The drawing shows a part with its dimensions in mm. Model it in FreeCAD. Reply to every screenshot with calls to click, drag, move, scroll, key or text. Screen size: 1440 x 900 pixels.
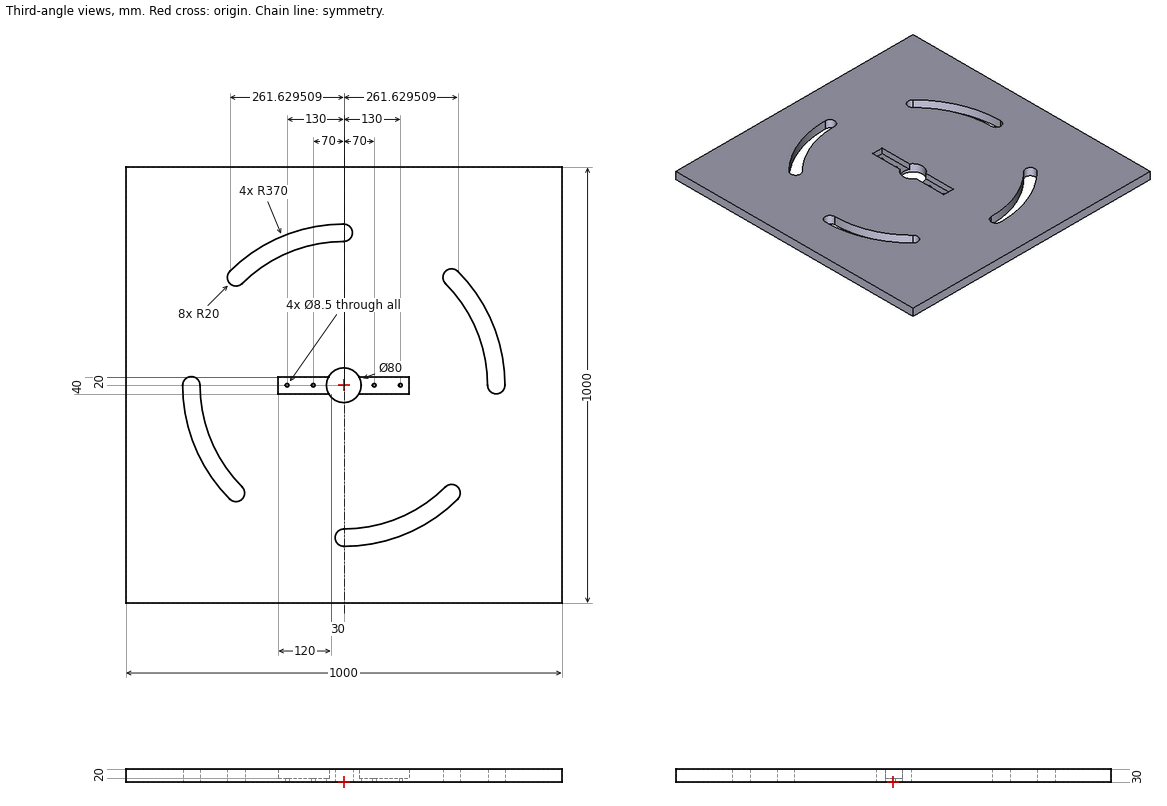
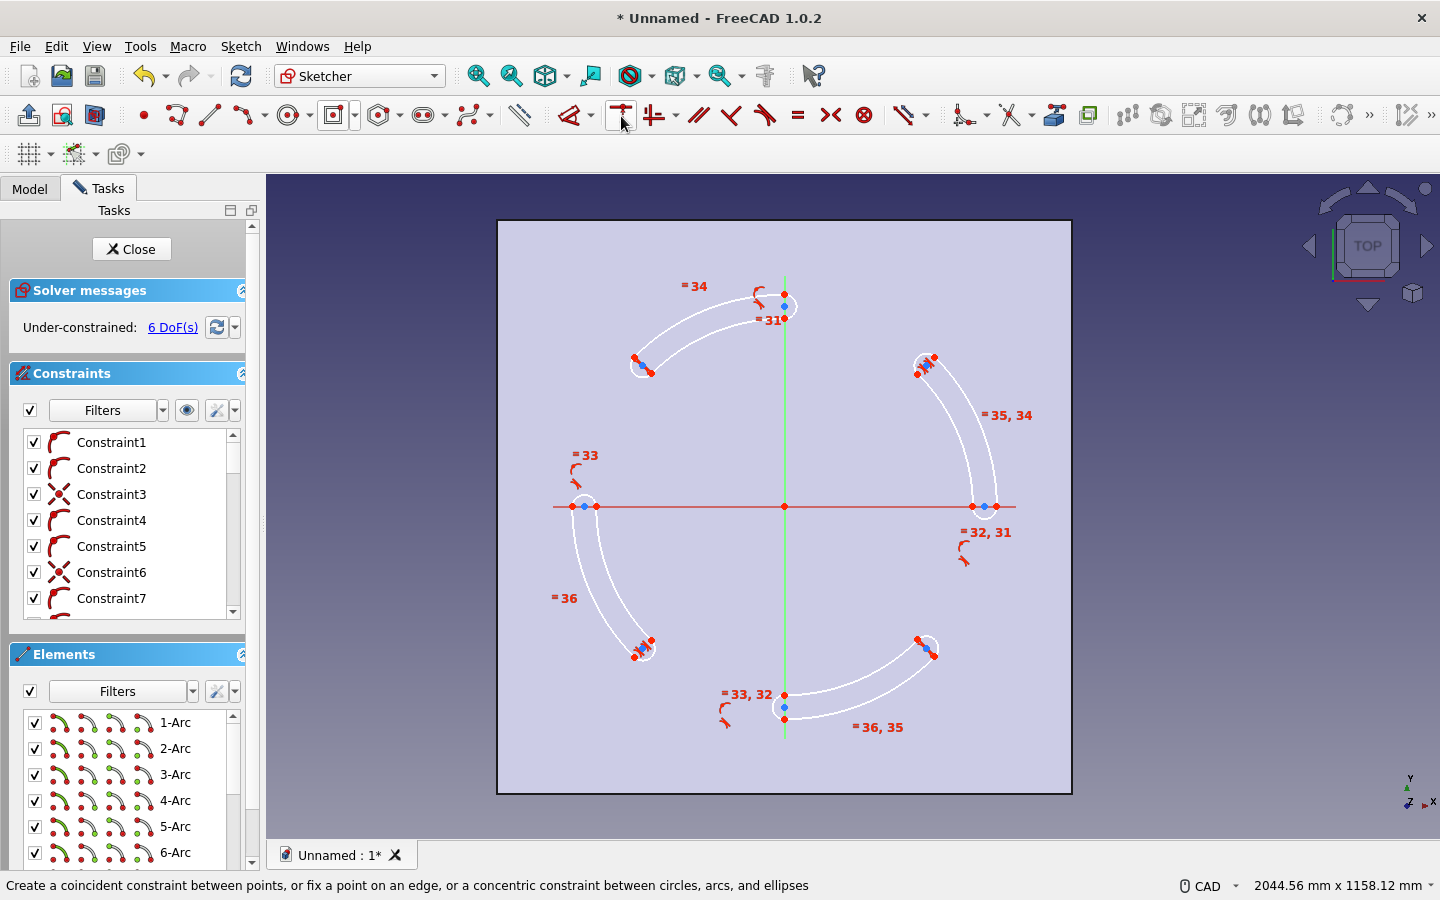
click(568, 116)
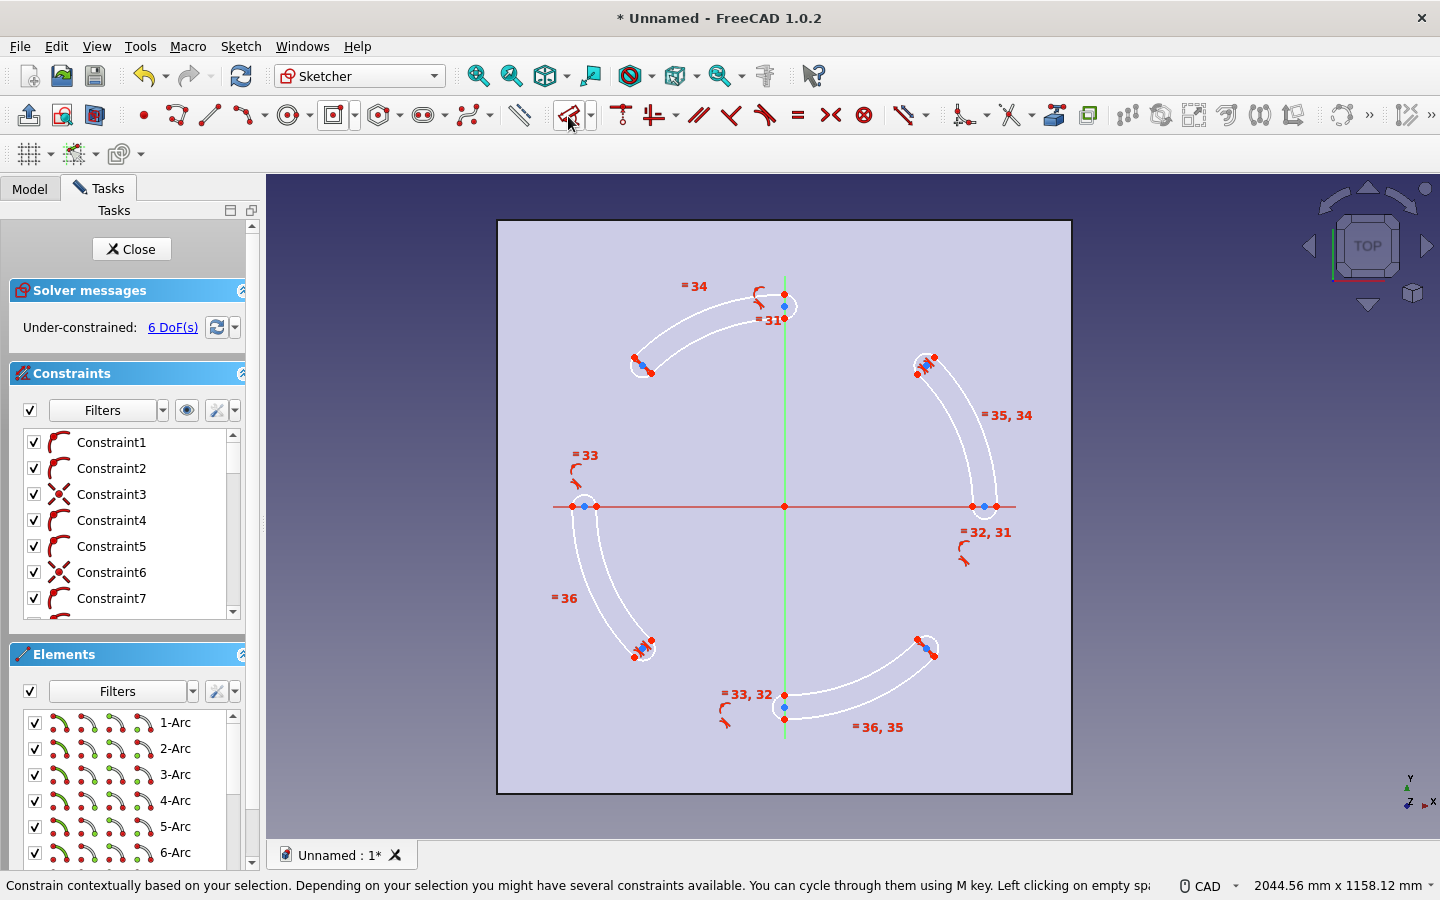
scroll(794, 314, up, 7)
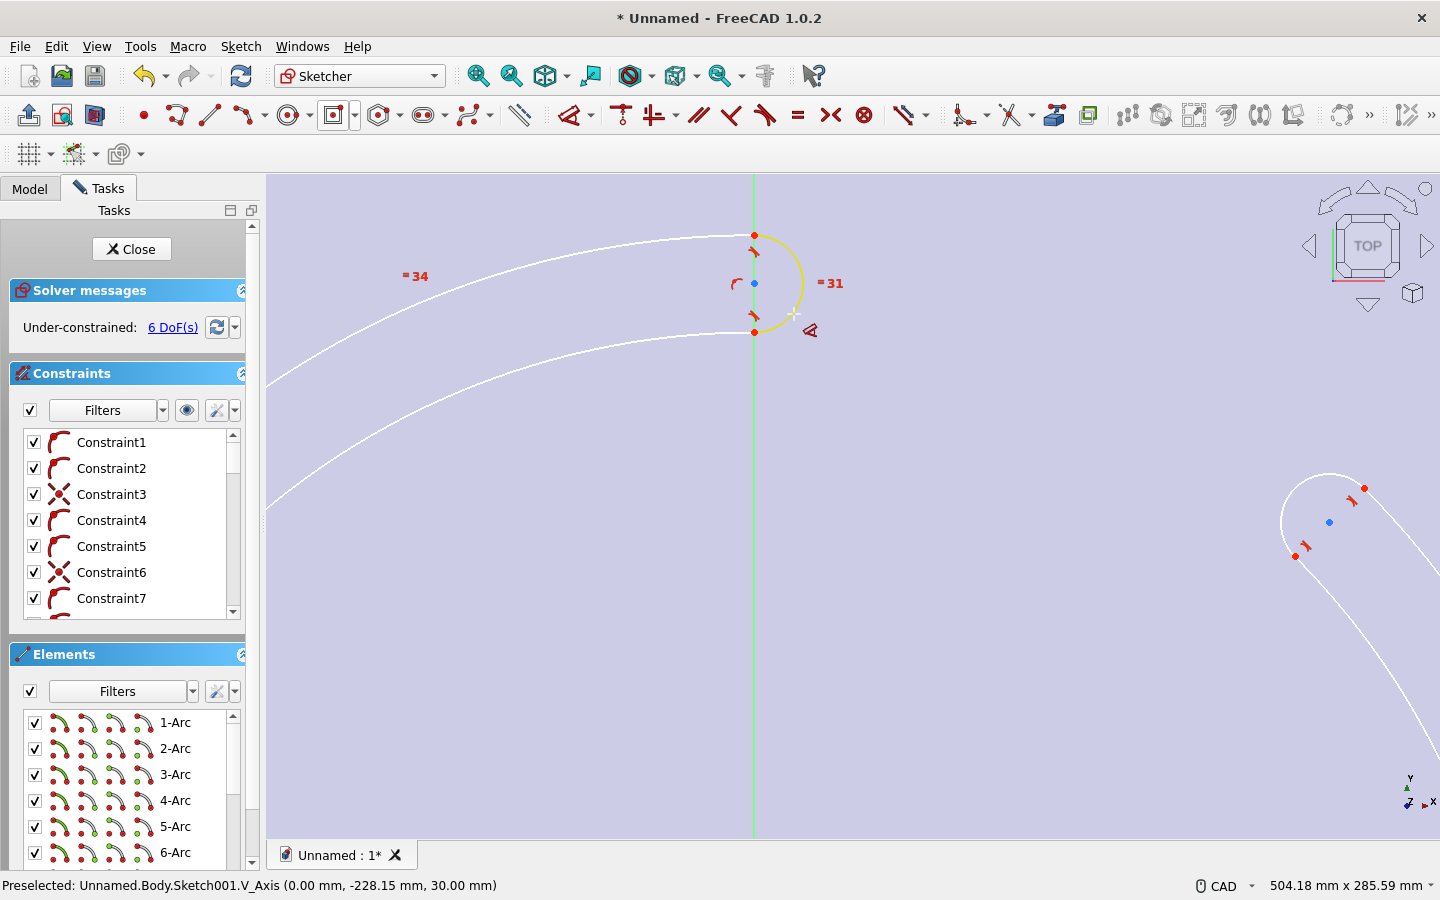
click(794, 312)
click(820, 331)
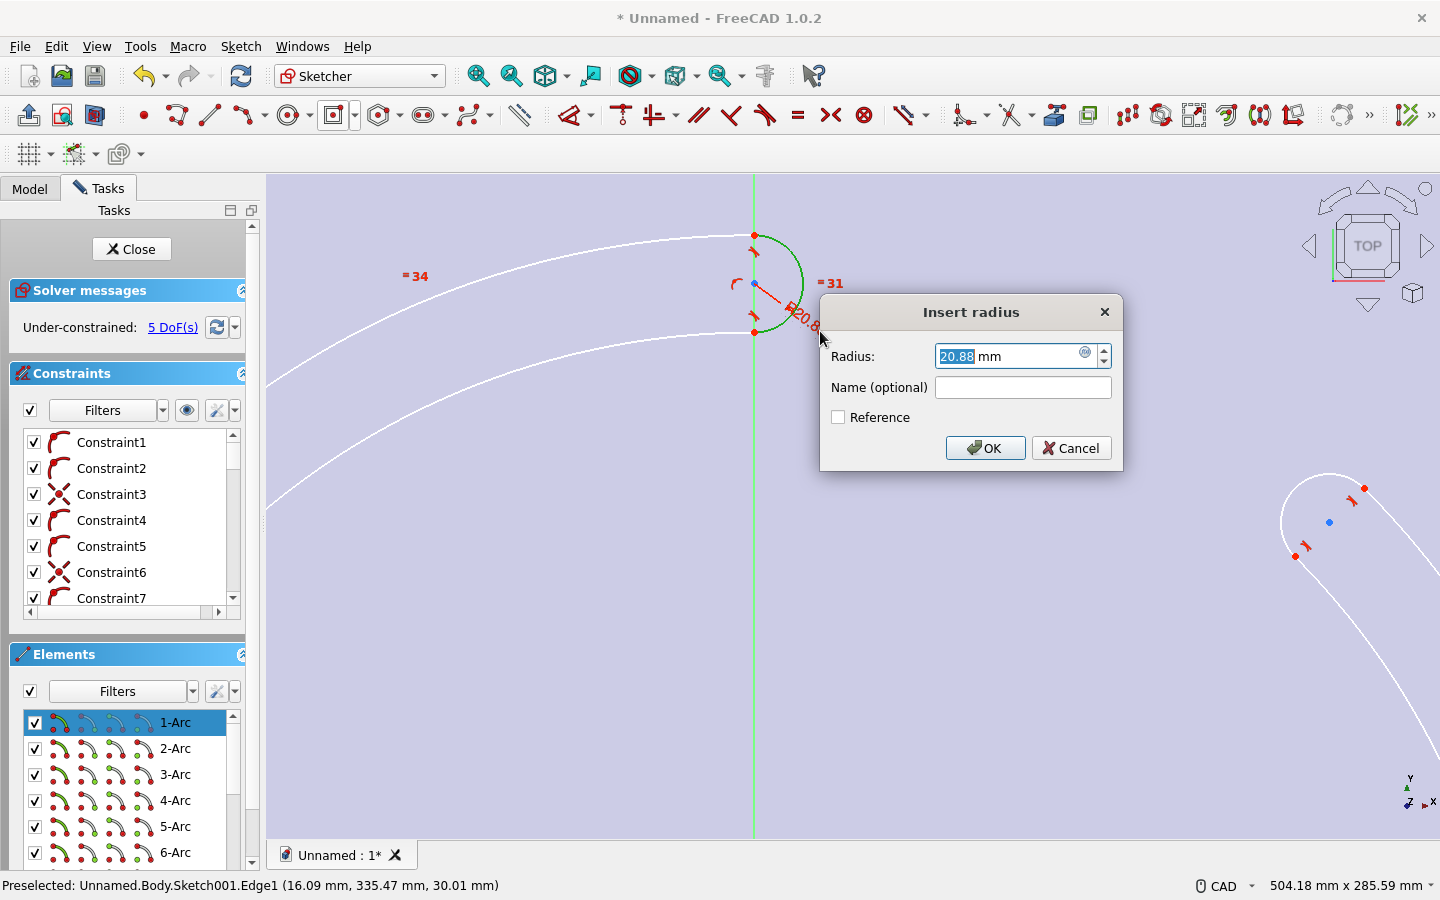
text(20)
key(Return)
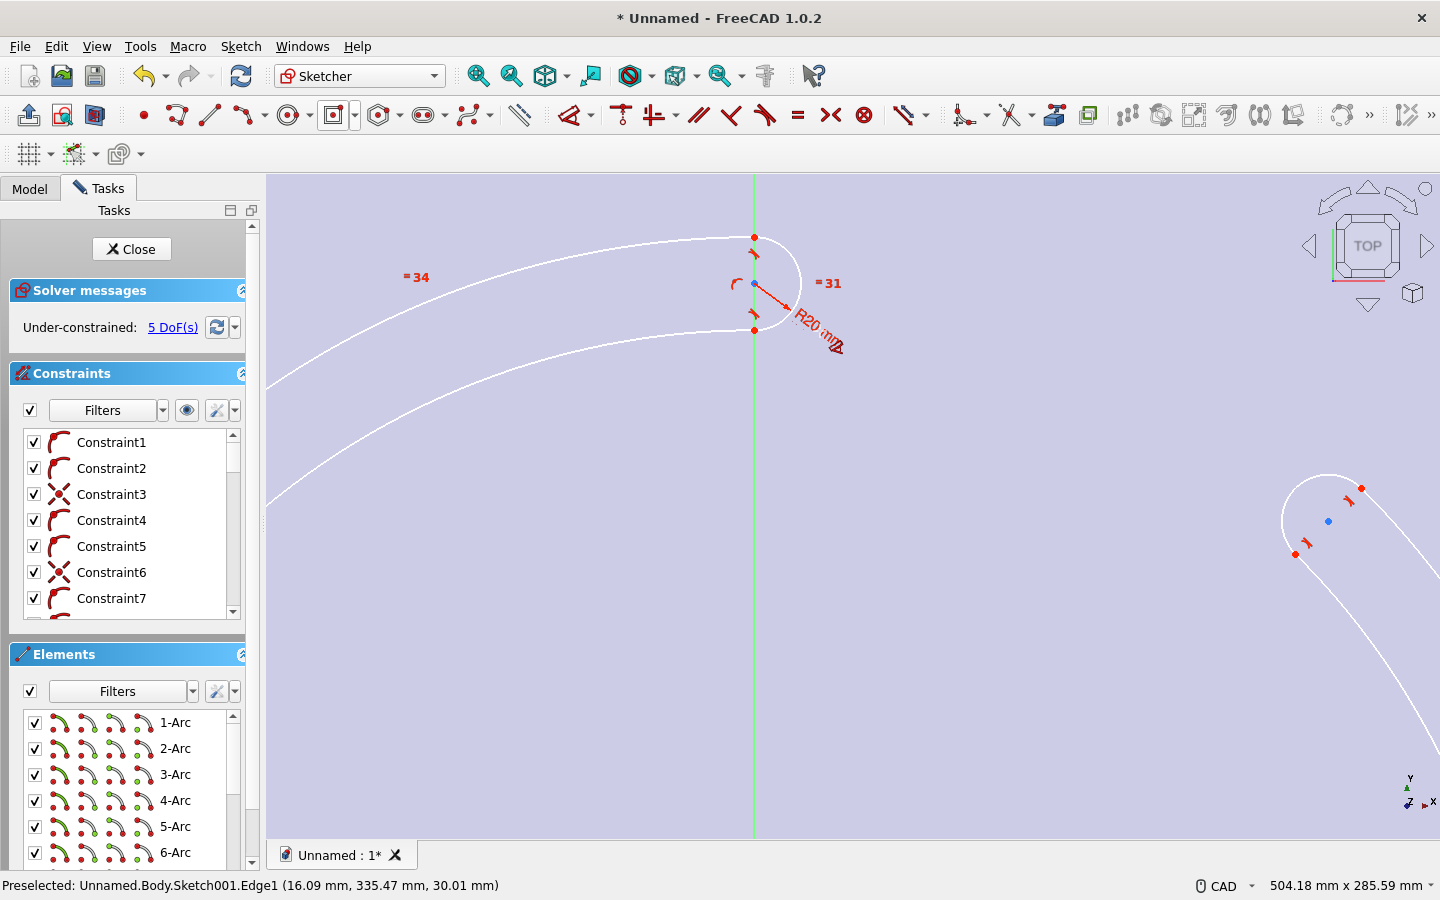
scroll(794, 314, down, 7)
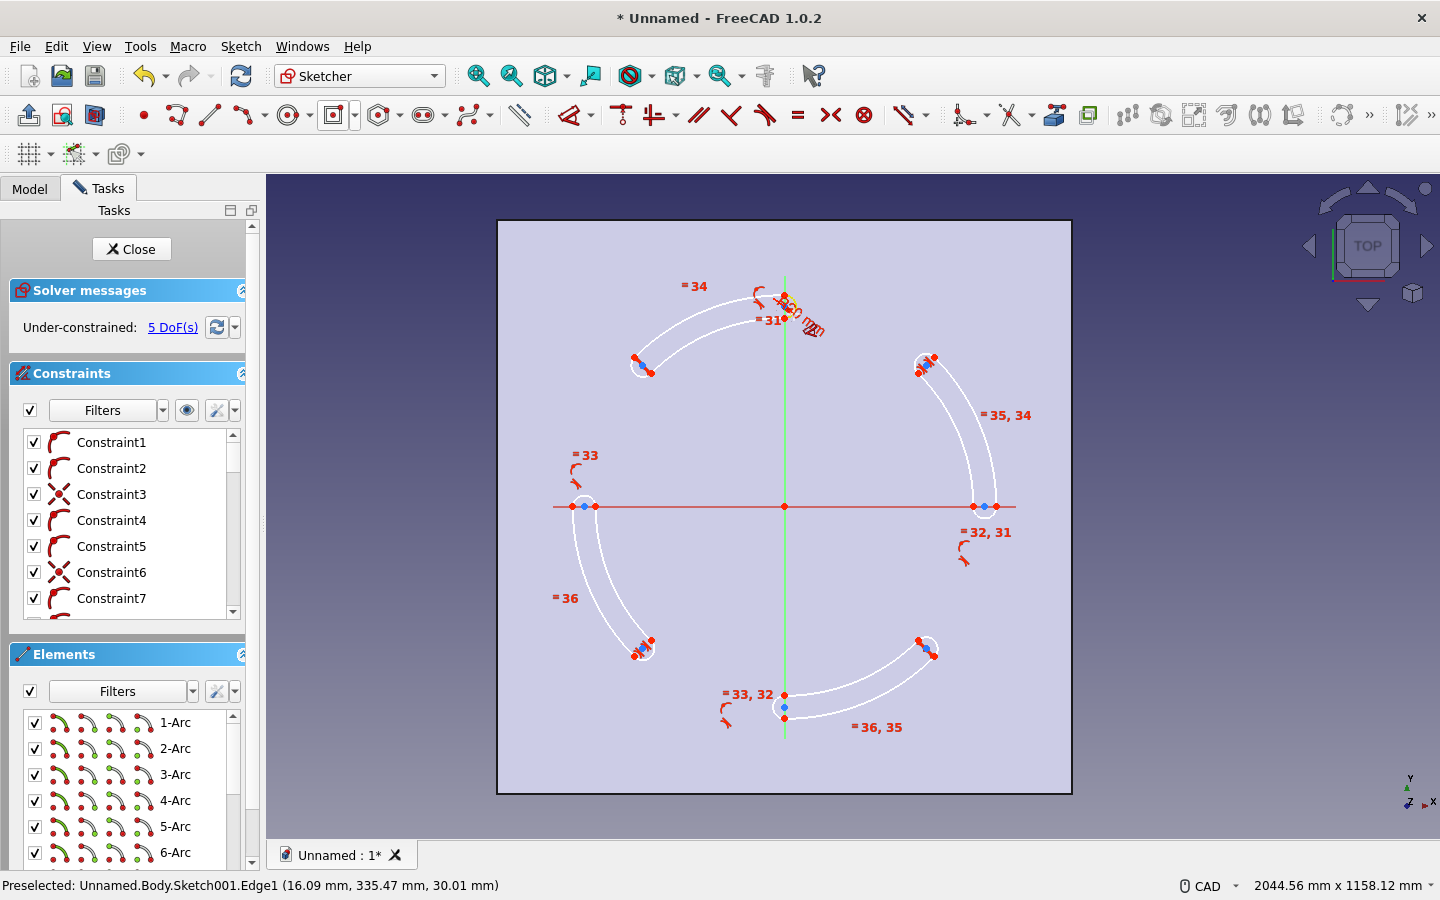
click(735, 301)
click(728, 270)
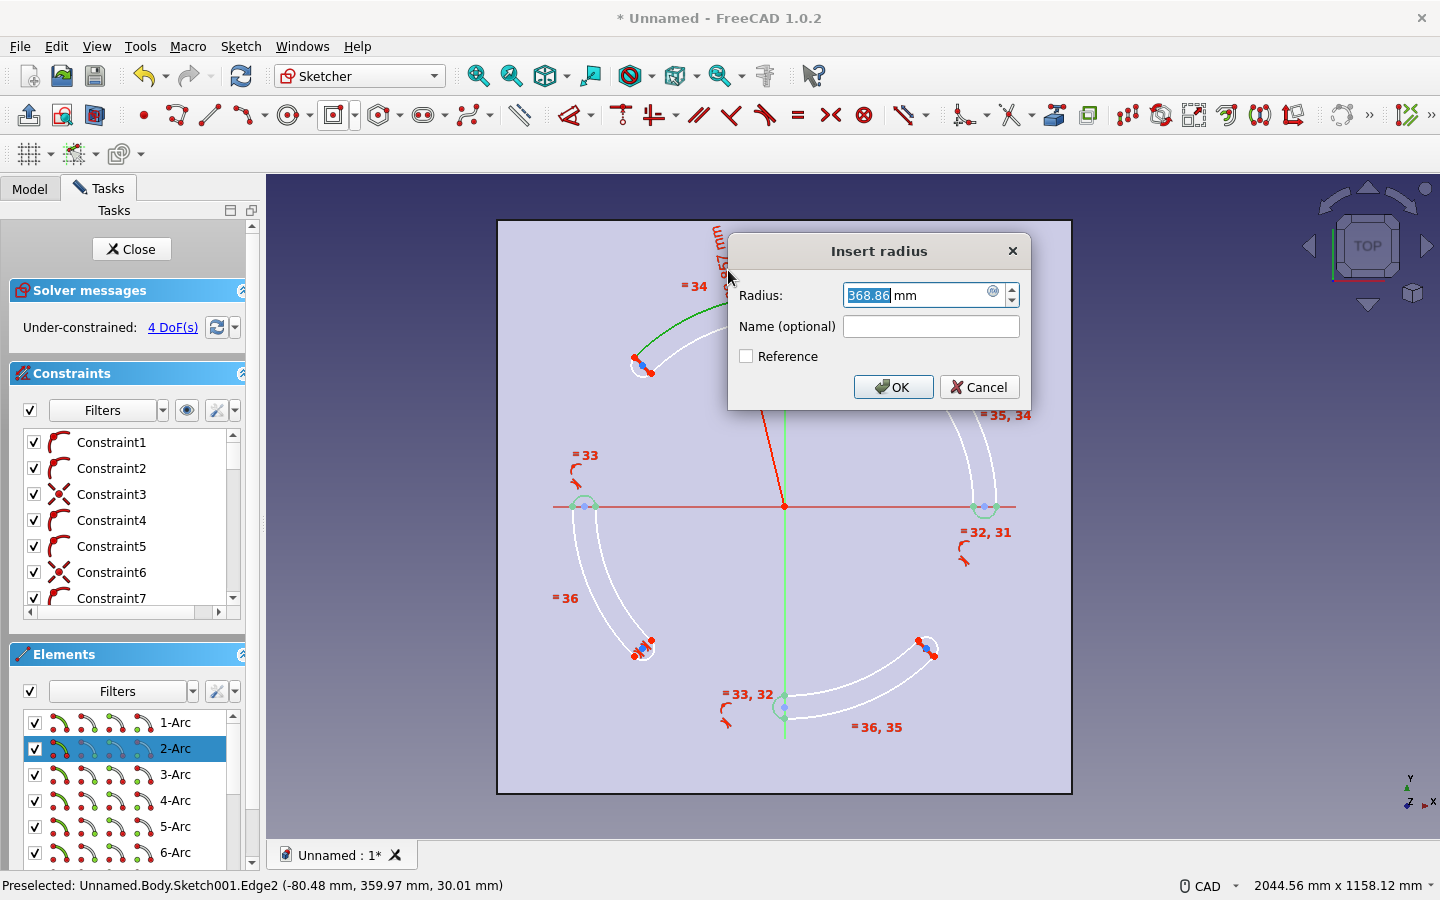
text(370)
key(Return)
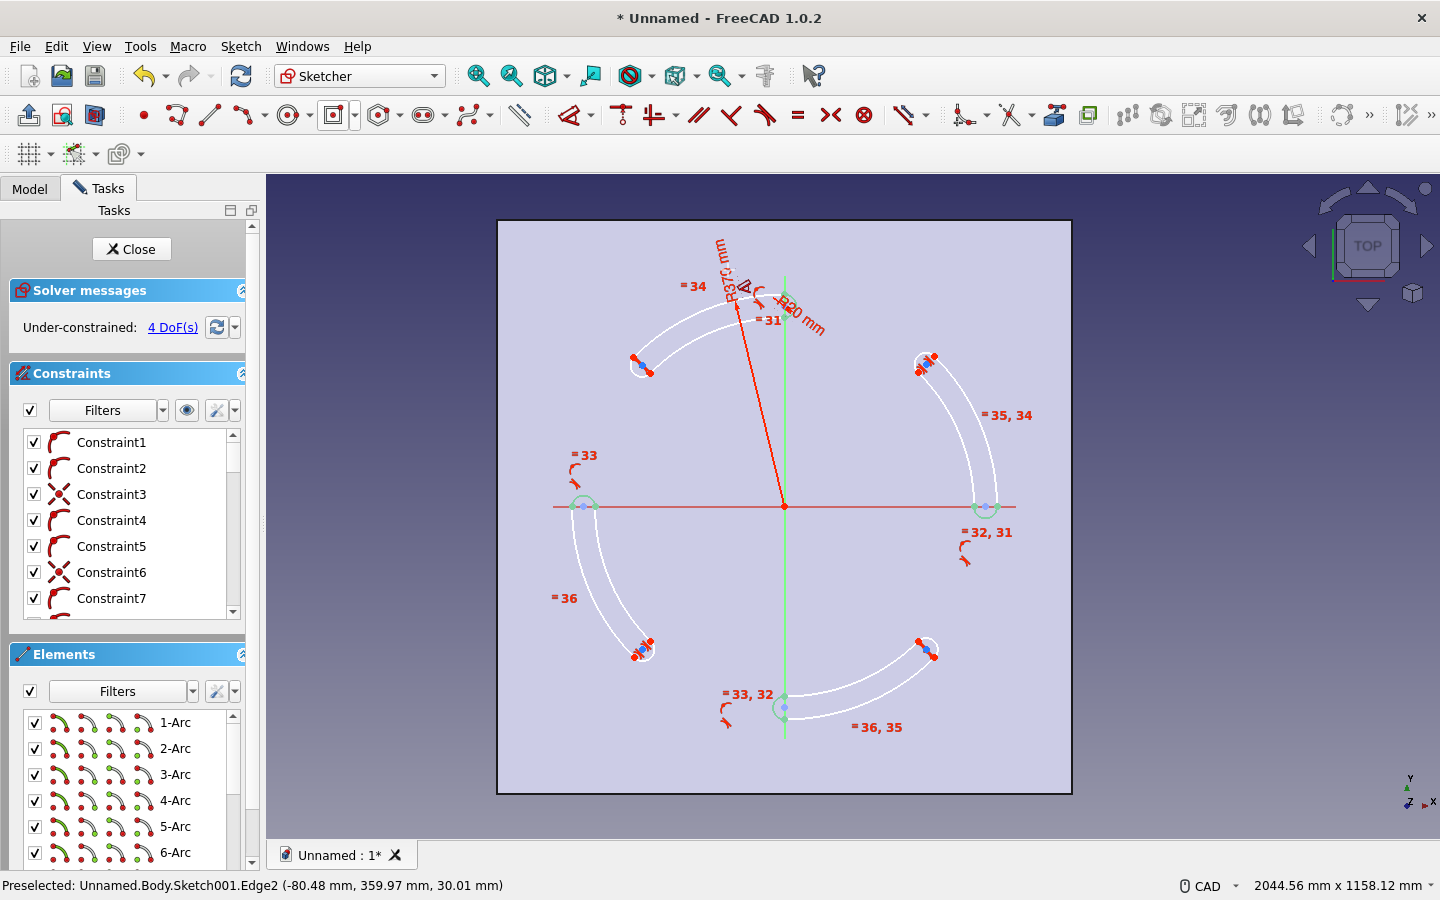
click(634, 357)
click(709, 541)